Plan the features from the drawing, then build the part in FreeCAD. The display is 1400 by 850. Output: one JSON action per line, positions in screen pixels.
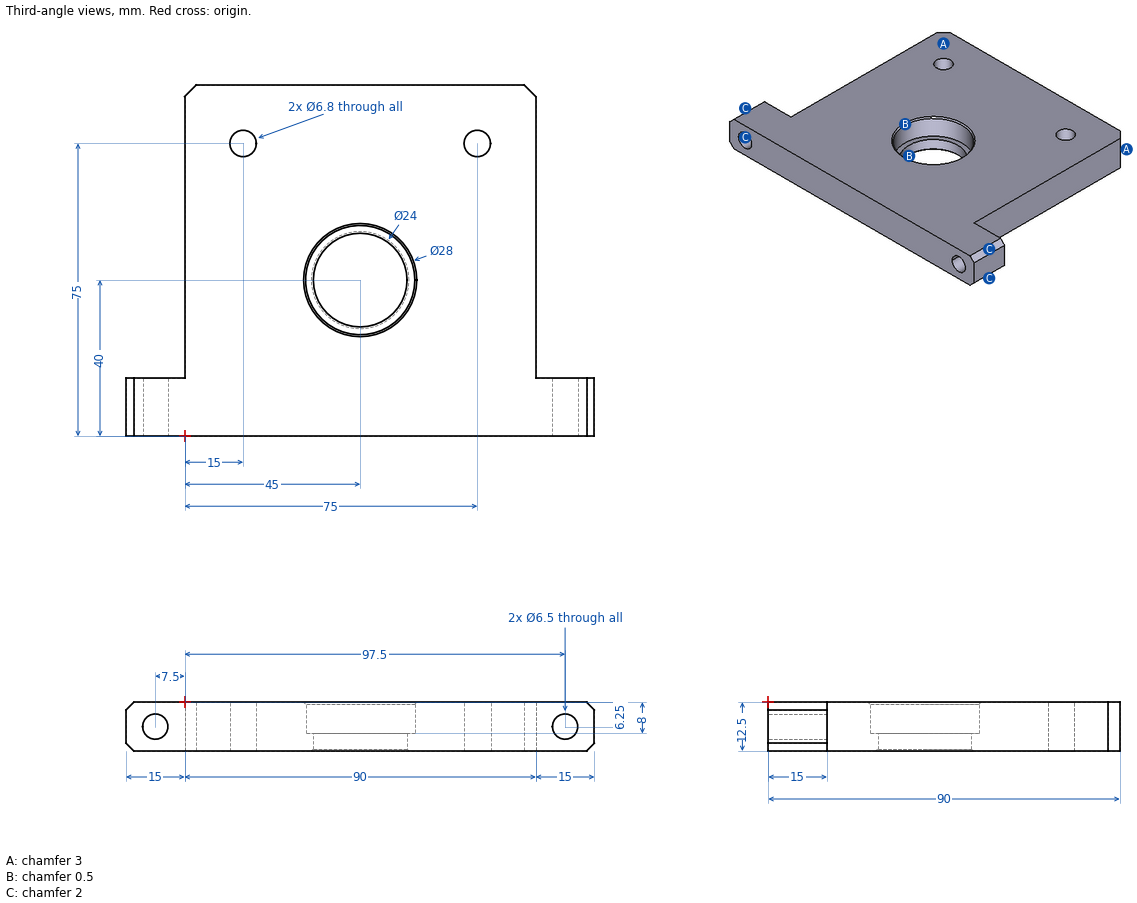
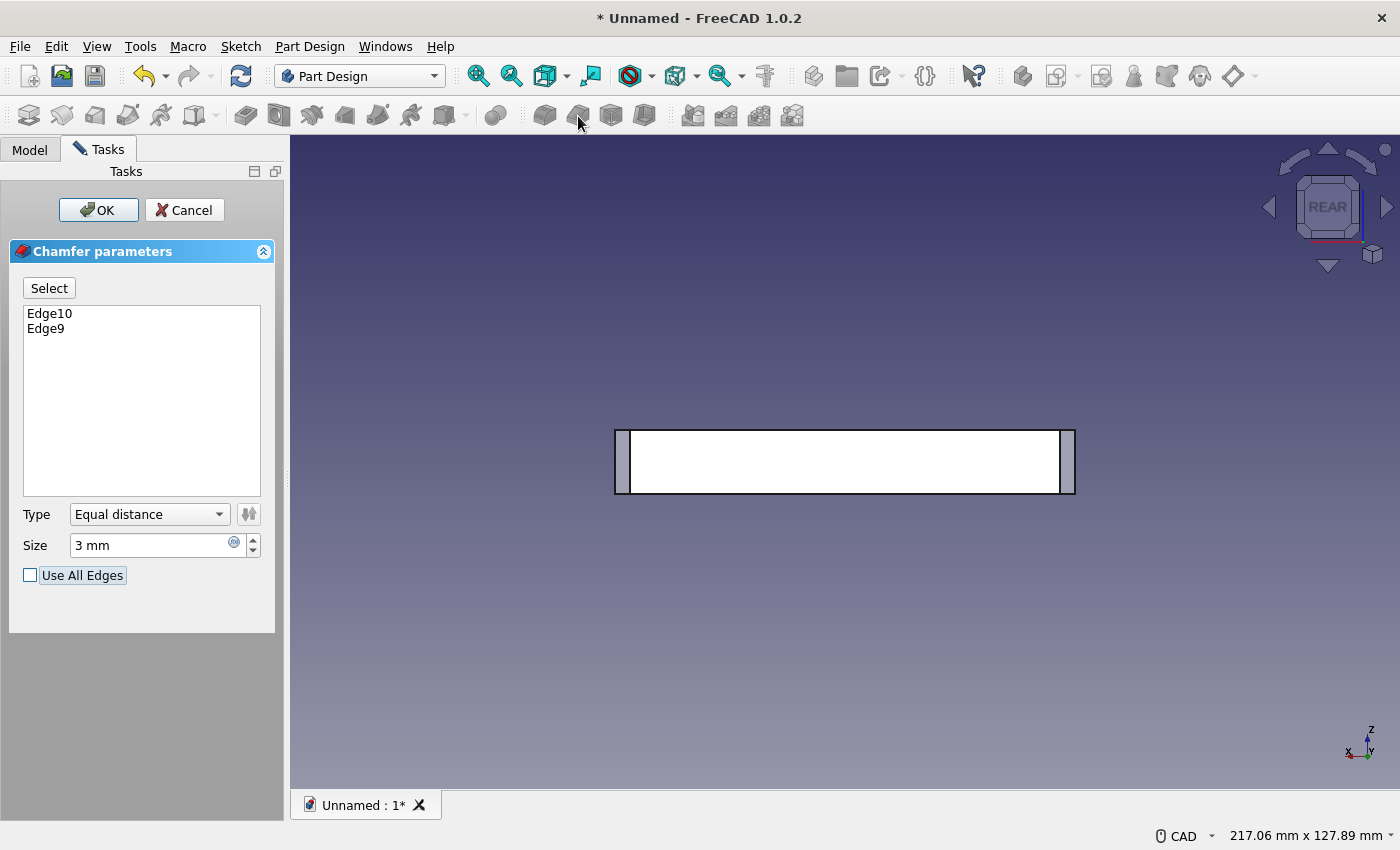
{"action": "left_click", "coordinate": [99, 210]}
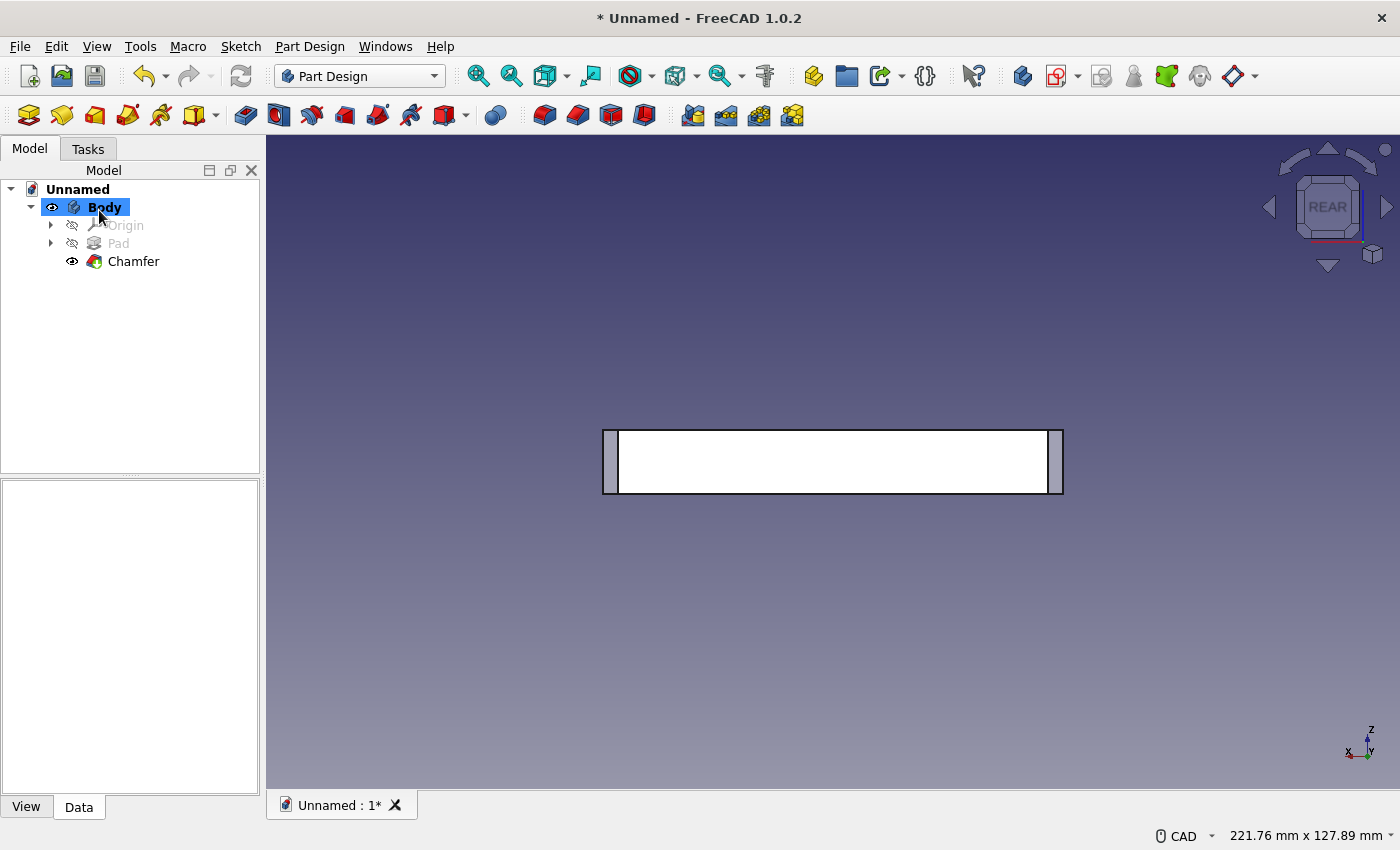
{"action": "left_click", "coordinate": [479, 76]}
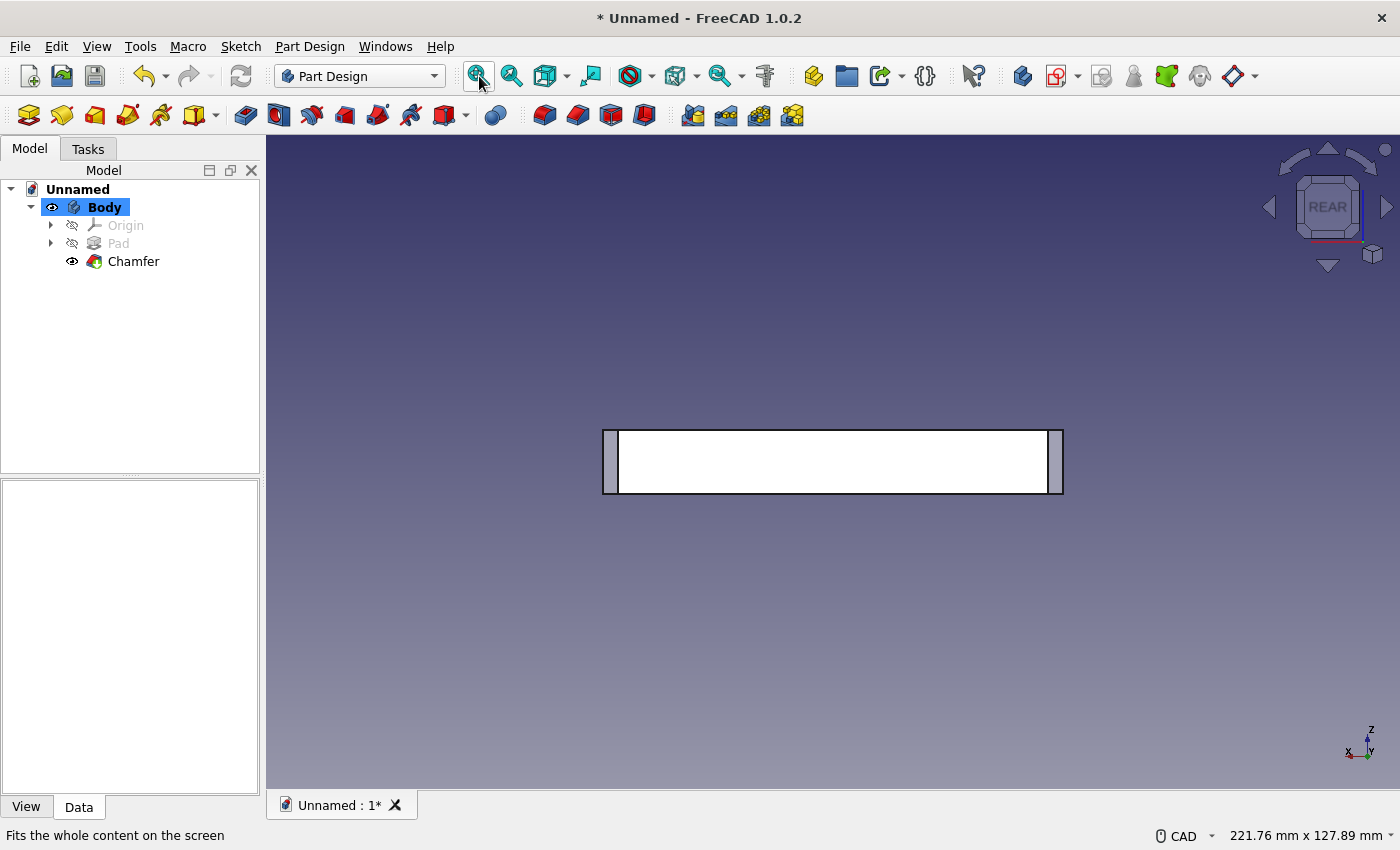
{"action": "key", "text": "5"}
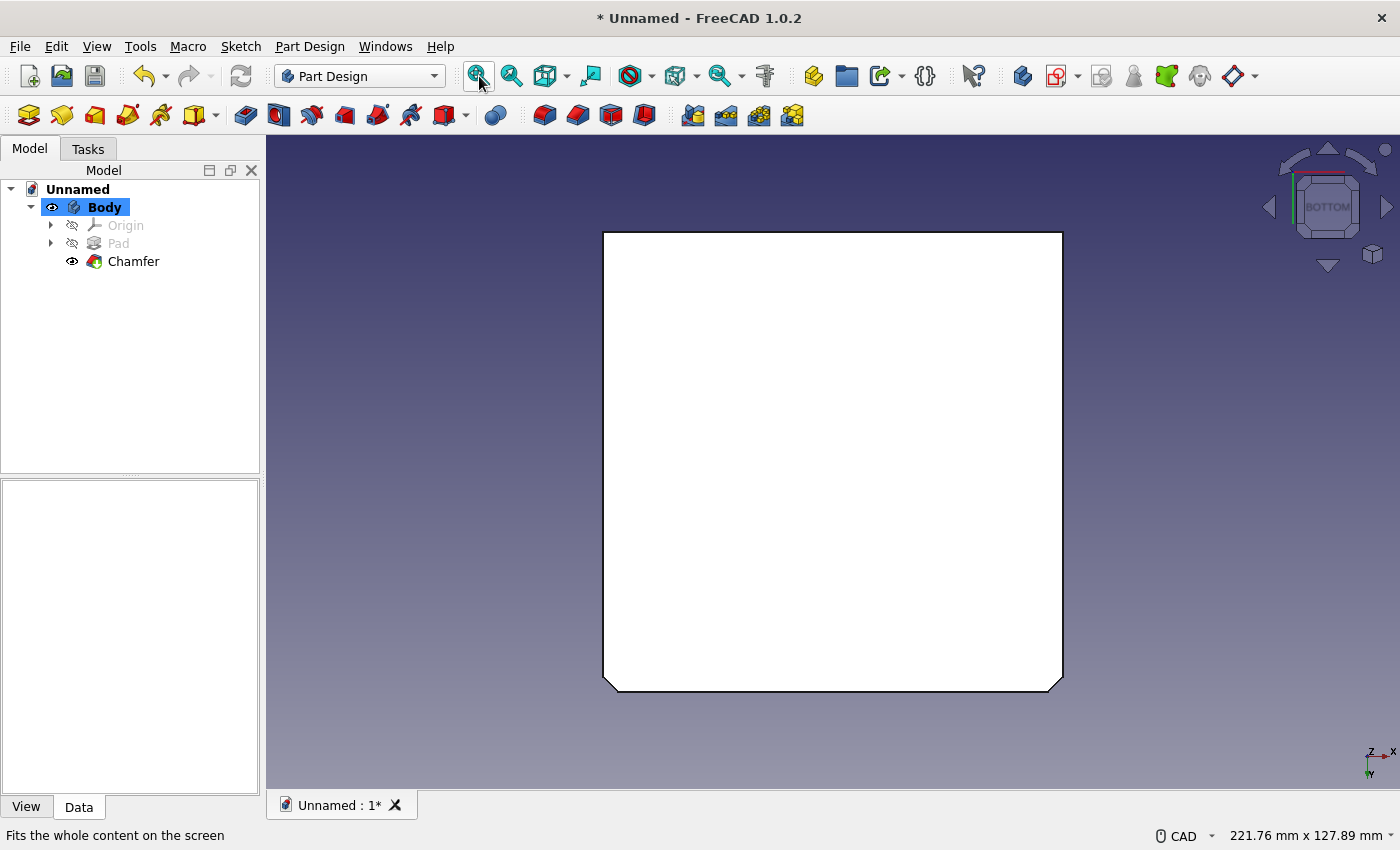
{"action": "left_click", "coordinate": [833, 461]}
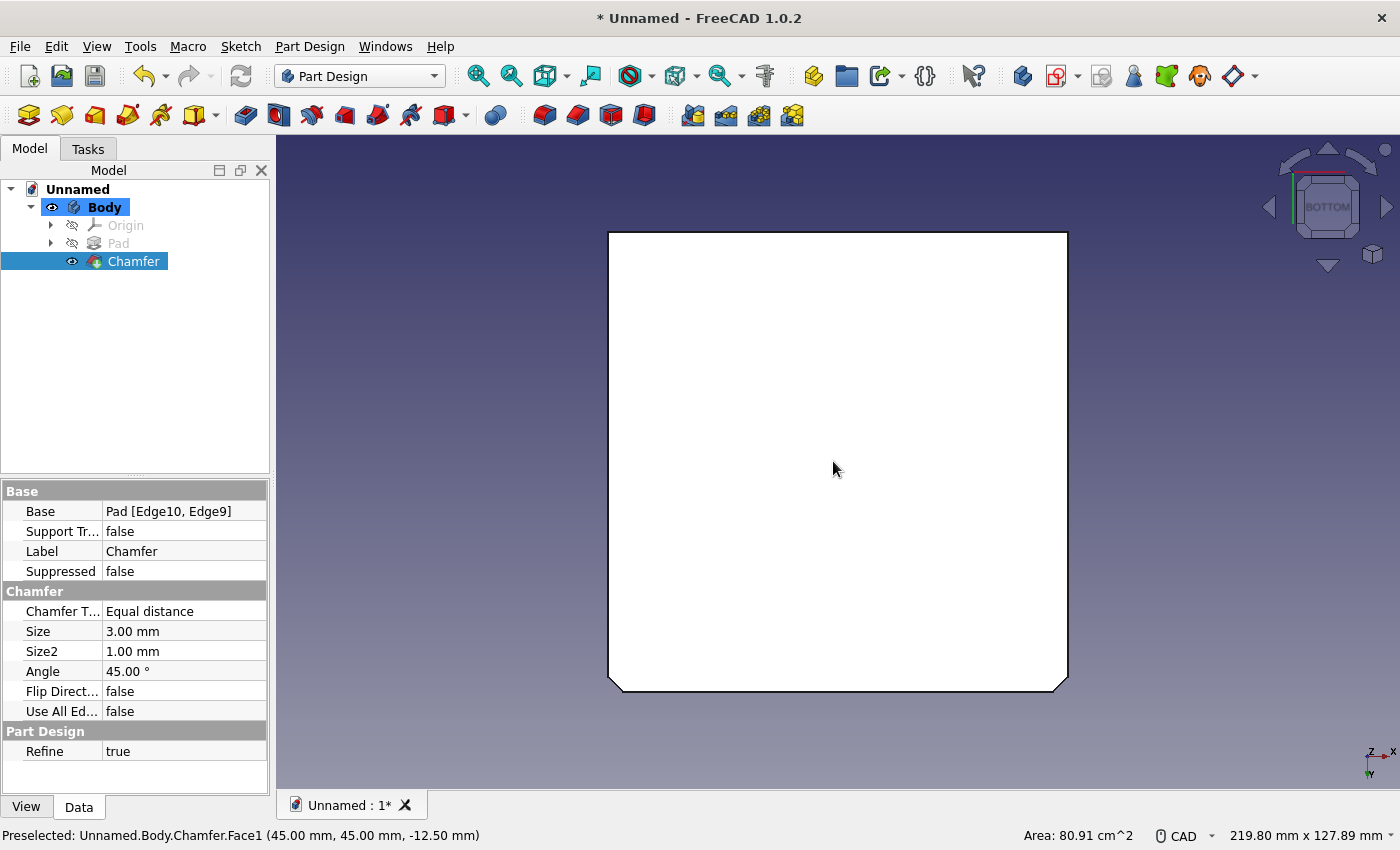
{"action": "left_click", "coordinate": [1056, 76]}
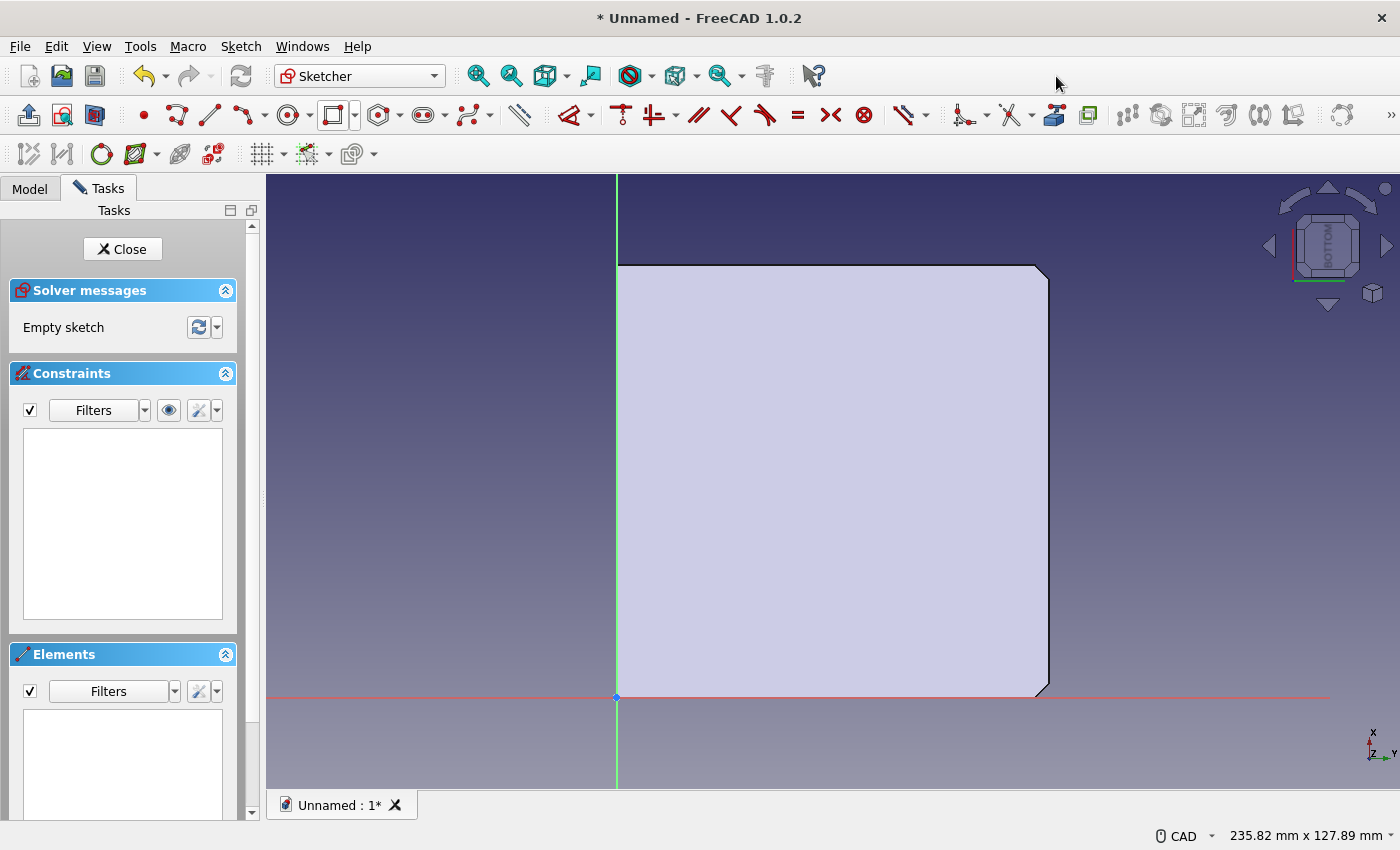
{"action": "left_click", "coordinate": [288, 116]}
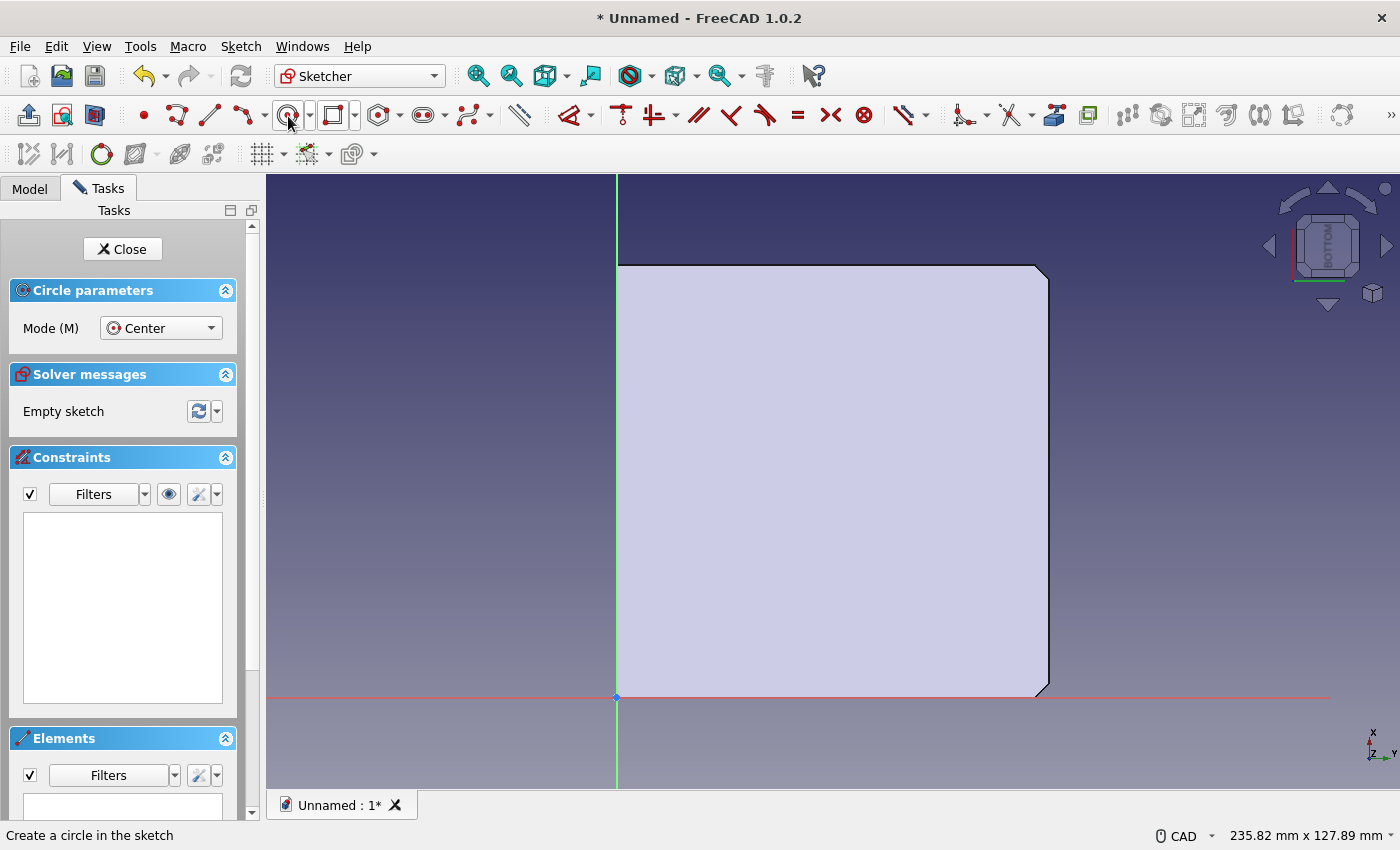
{"action": "scroll", "coordinate": [977, 626], "scroll_direction": "up", "scroll_amount": 2}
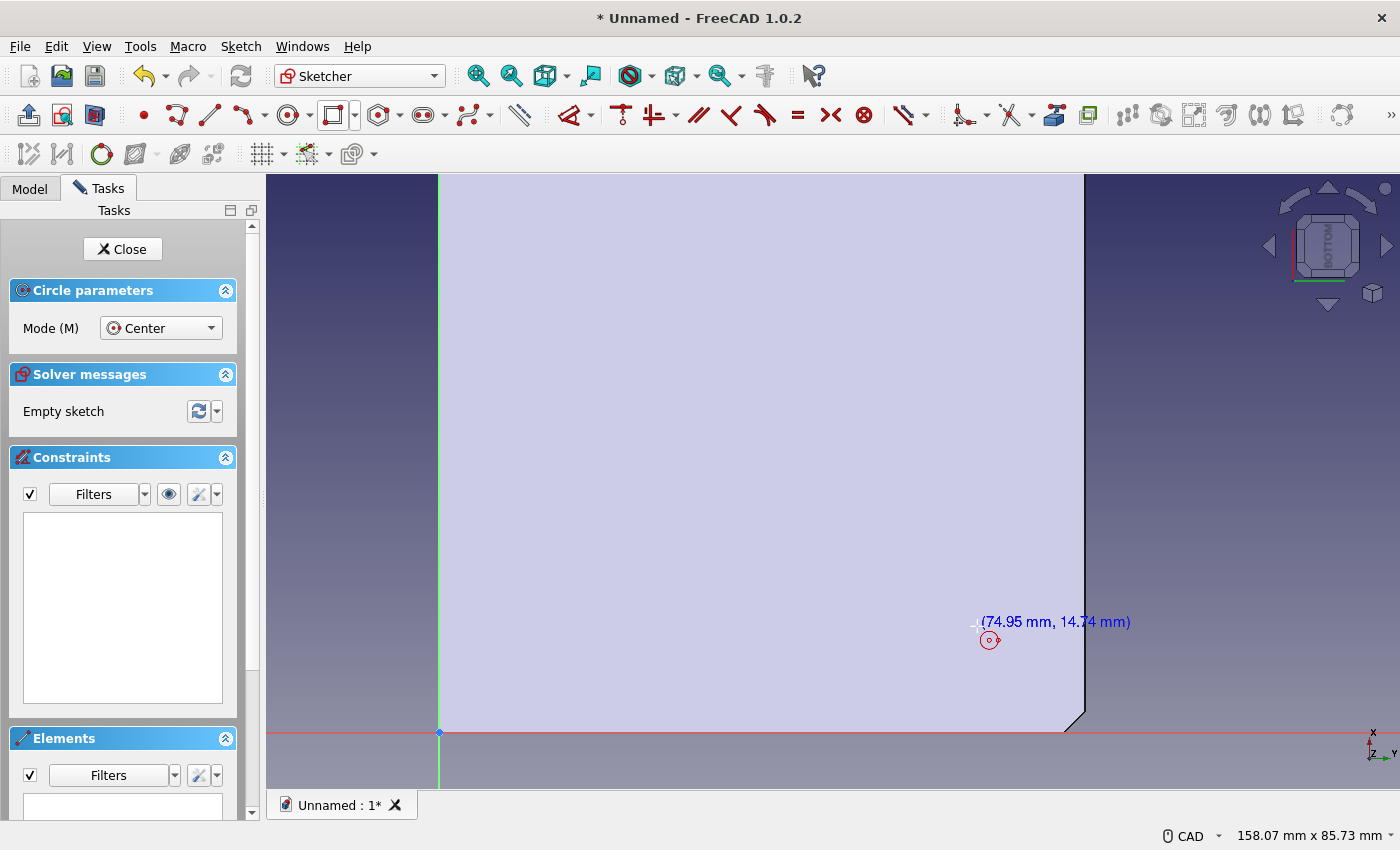
{"action": "left_click", "coordinate": [977, 625]}
{"action": "left_click", "coordinate": [994, 608]}